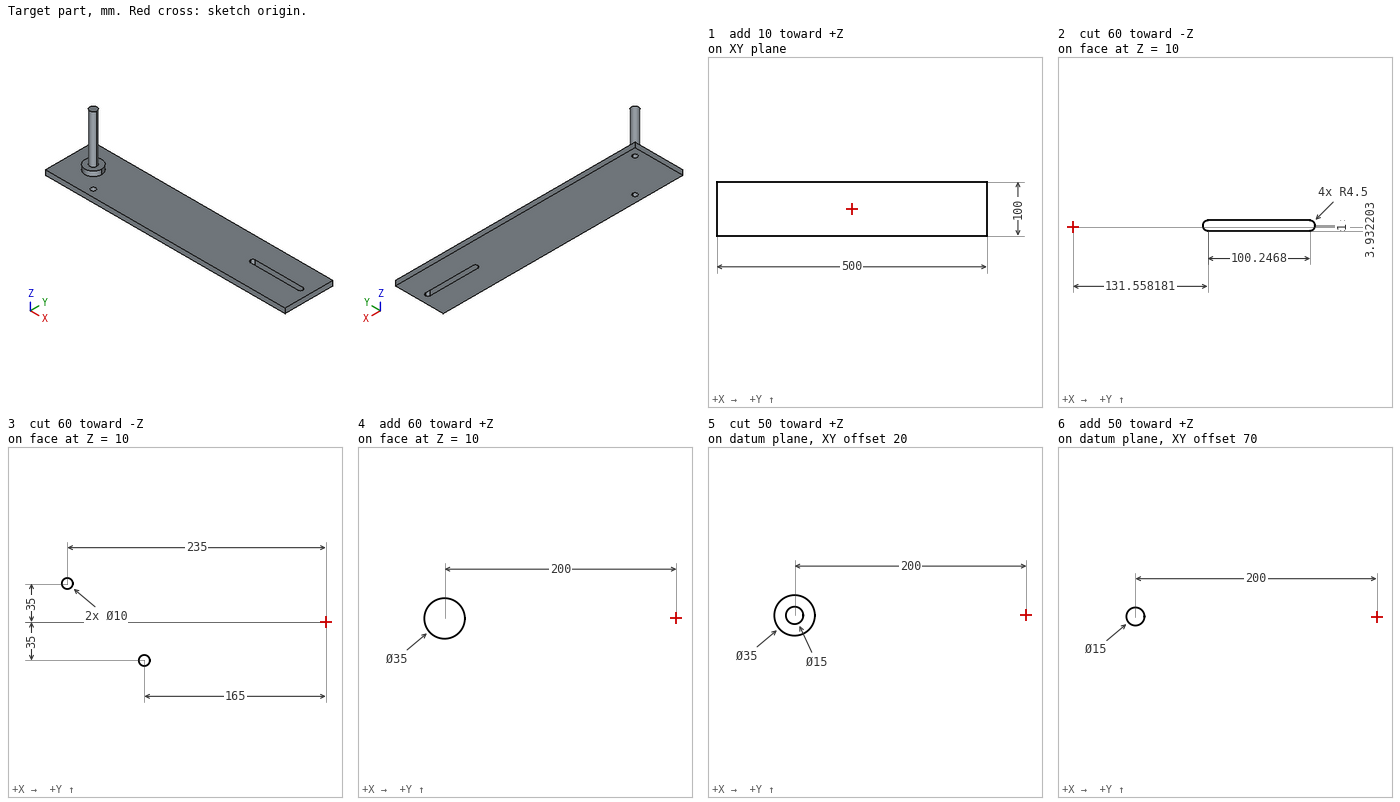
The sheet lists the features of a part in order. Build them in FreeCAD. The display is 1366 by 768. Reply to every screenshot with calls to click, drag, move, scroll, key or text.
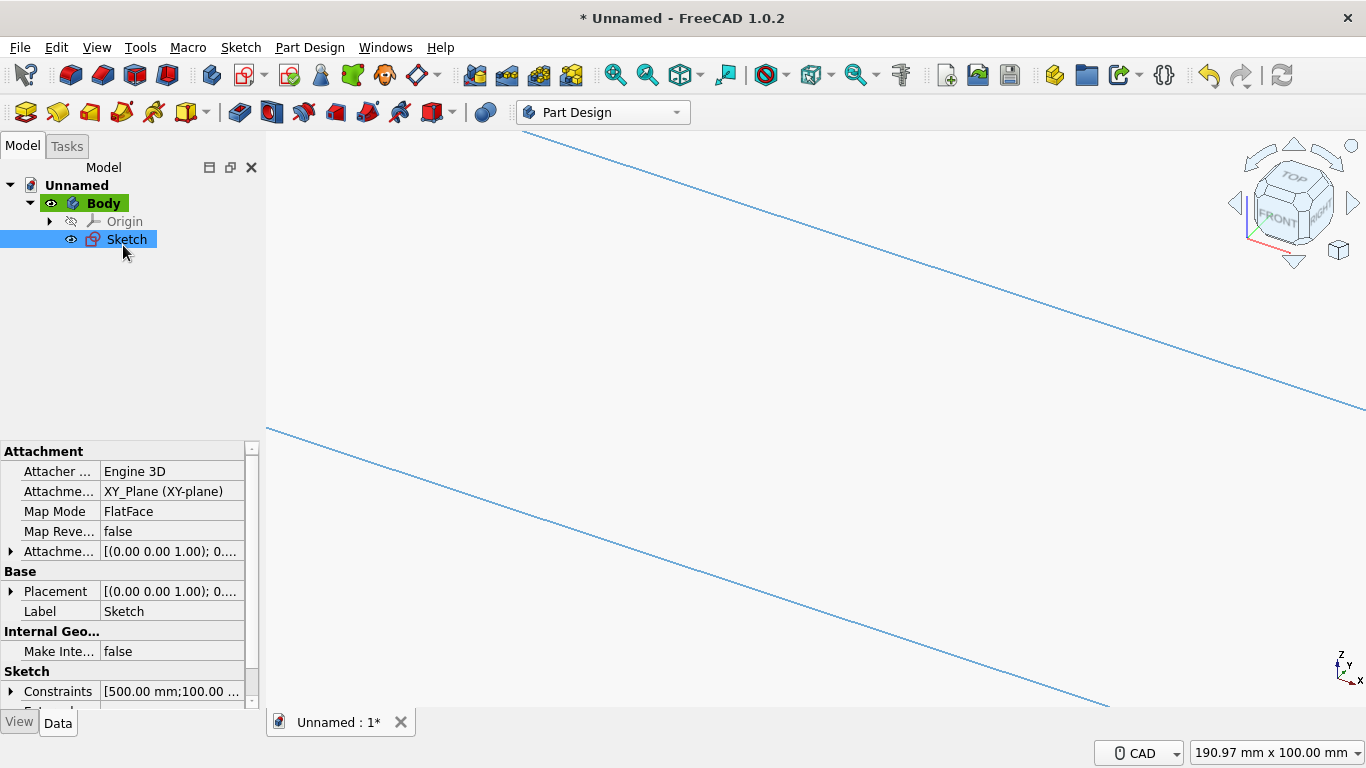
click(26, 112)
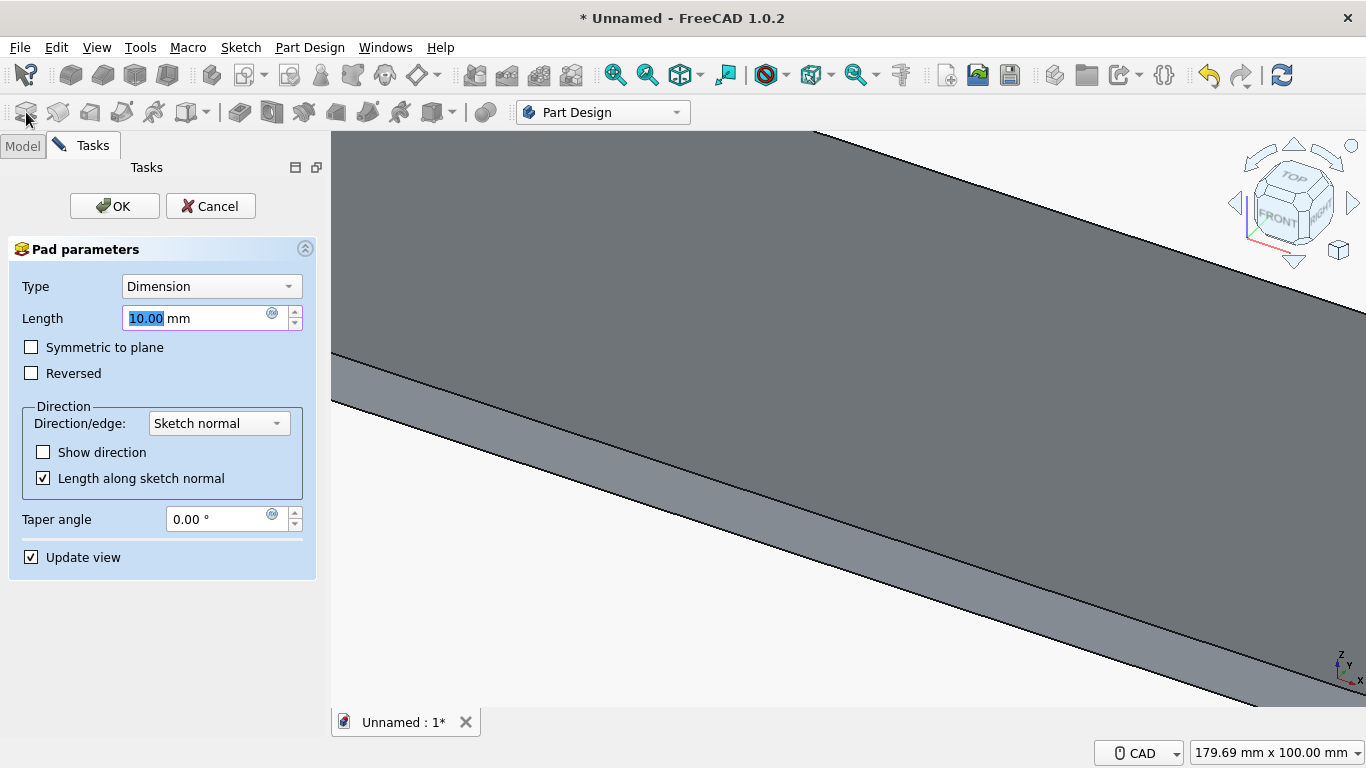
text(10)
key(Tab)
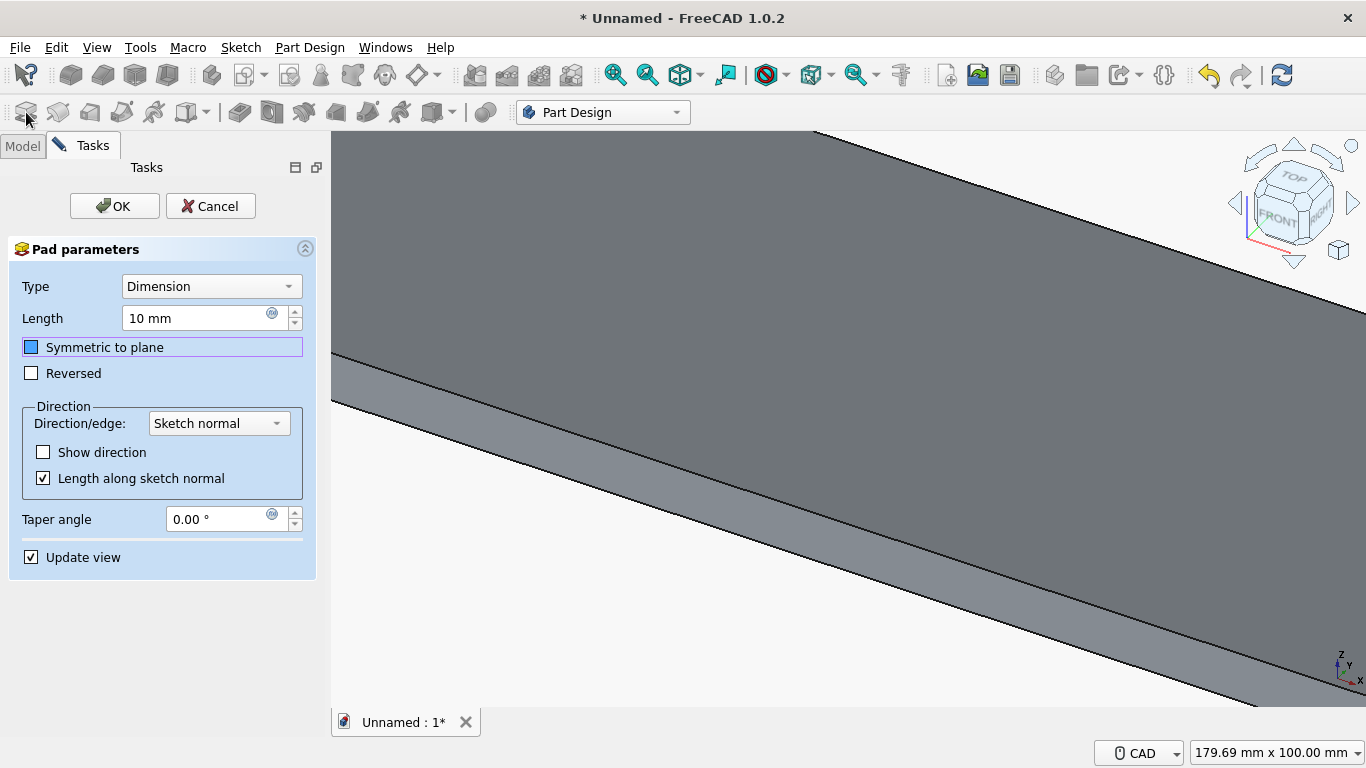
click(115, 206)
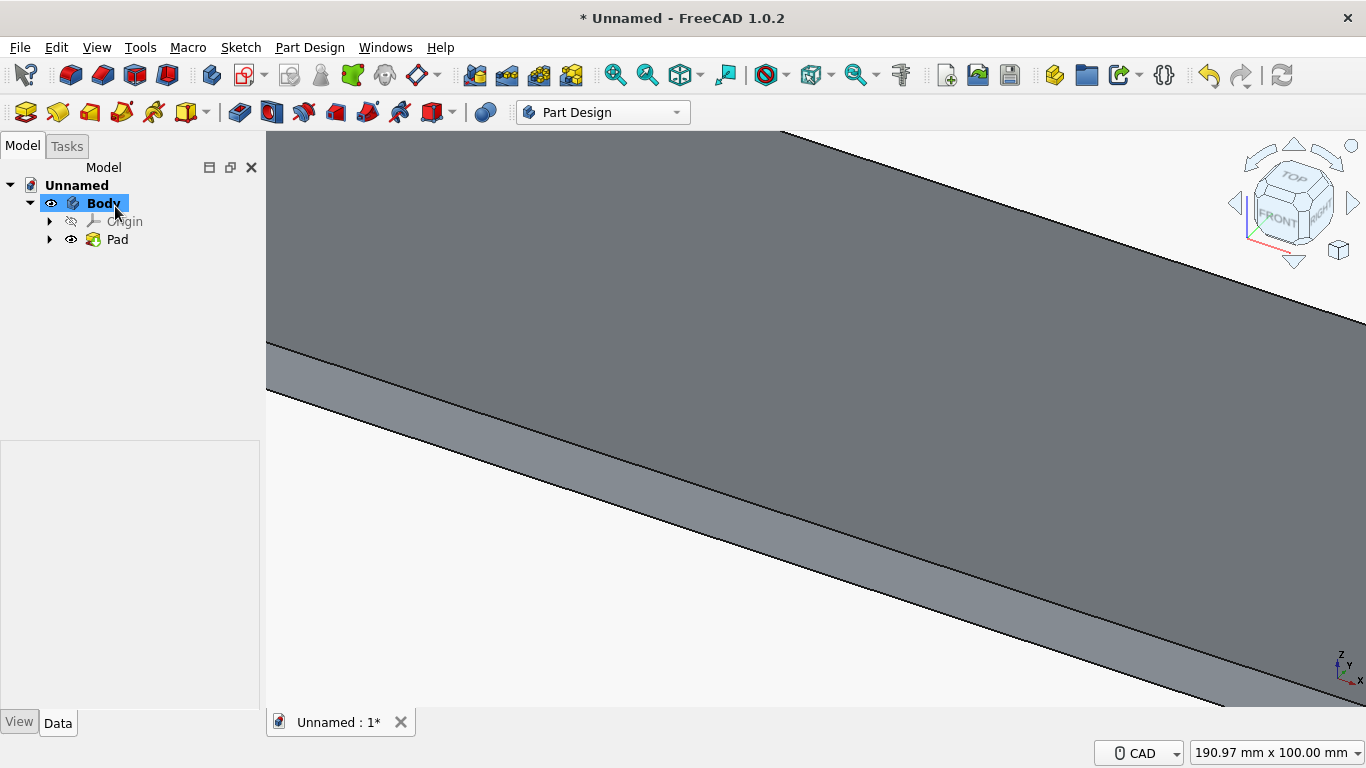
key(v)
key(f)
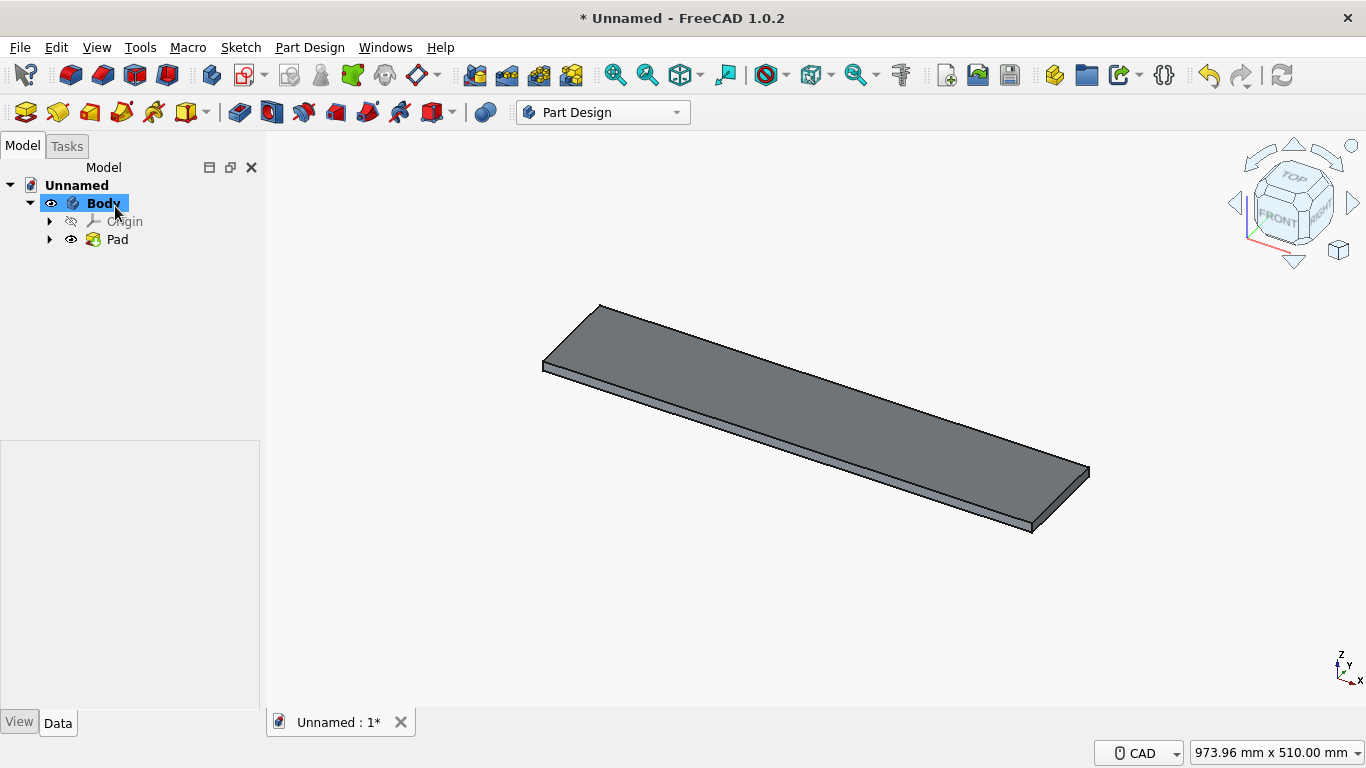
click(956, 460)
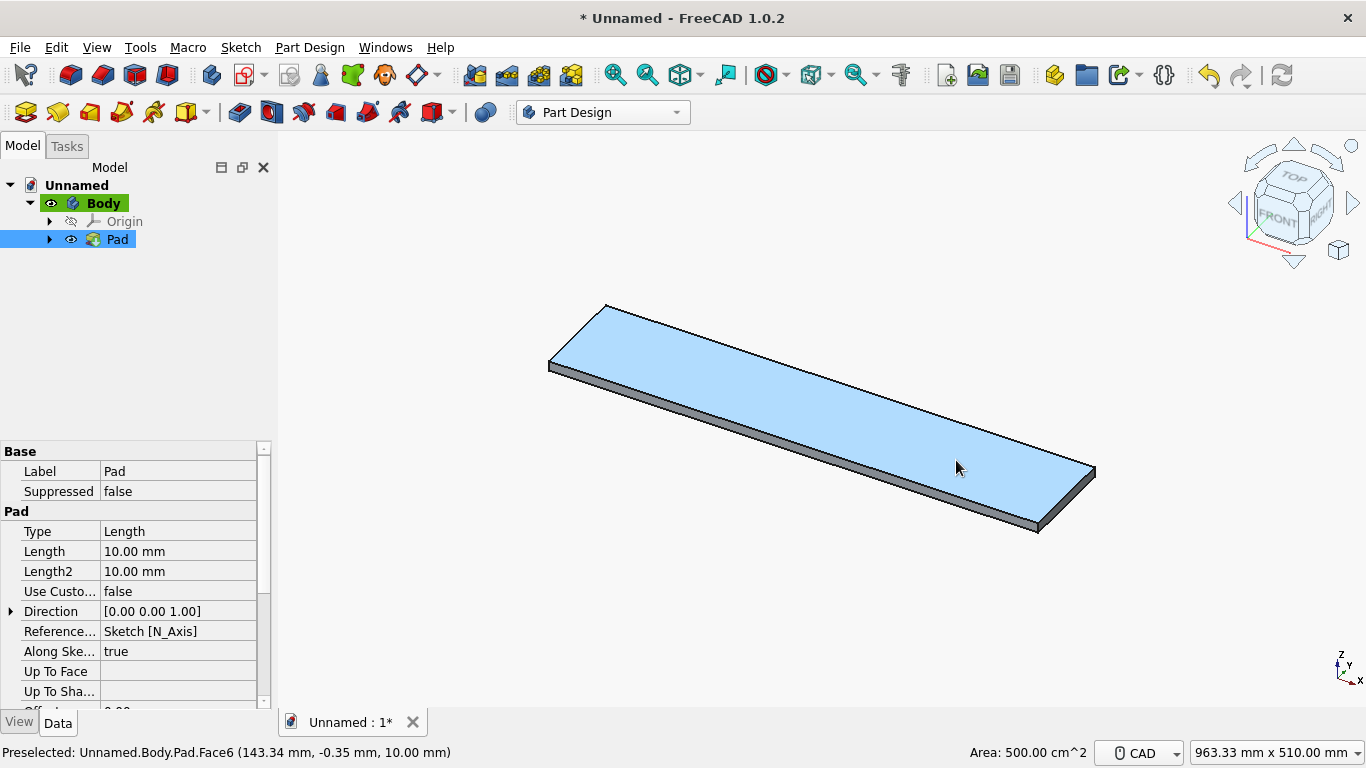
click(244, 76)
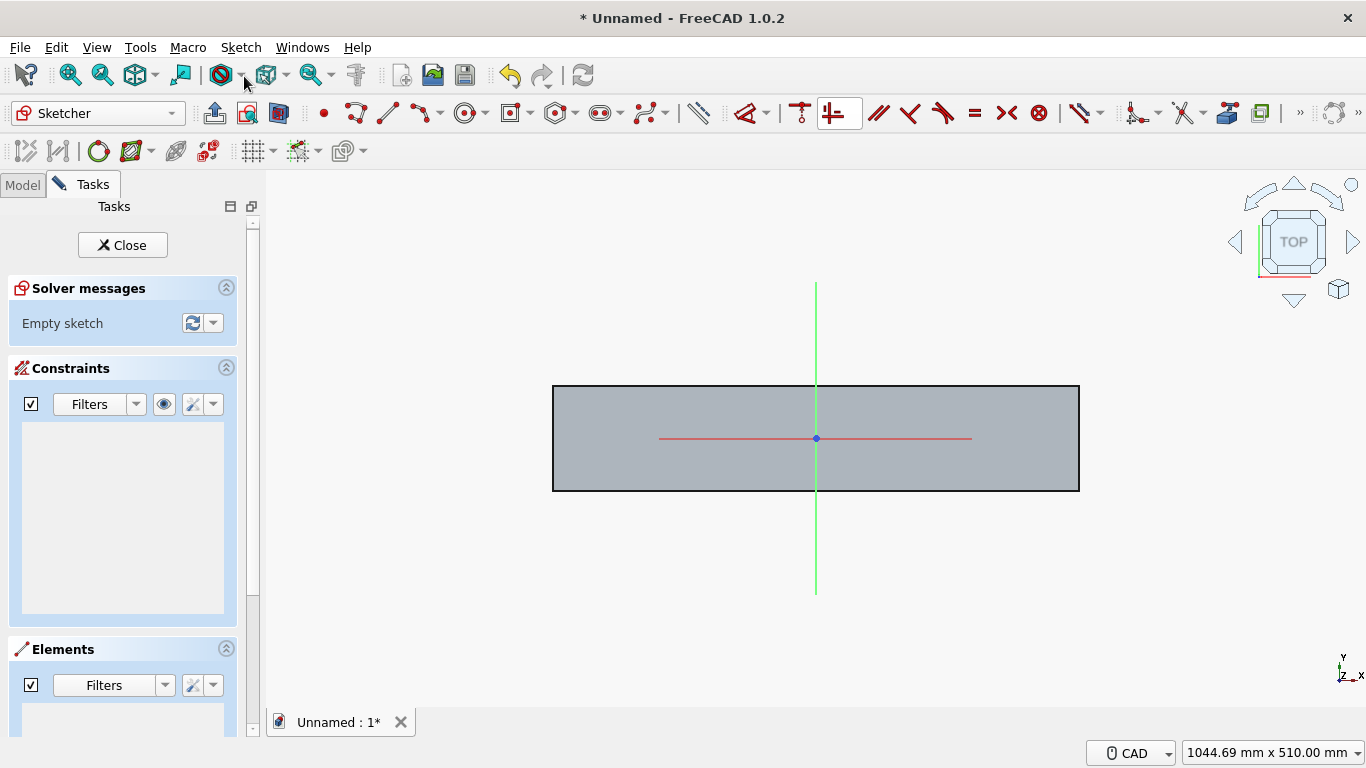
scroll(1053, 437, up, 5)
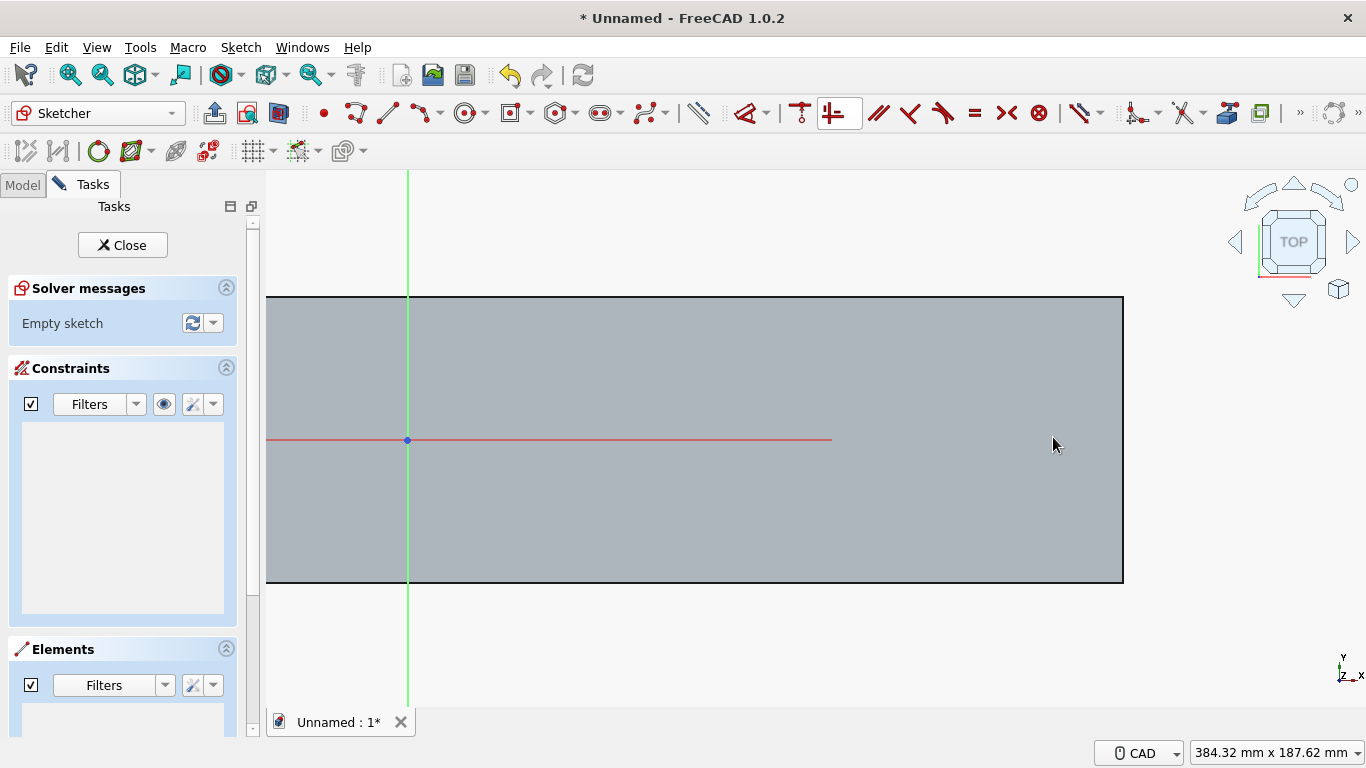
click(388, 114)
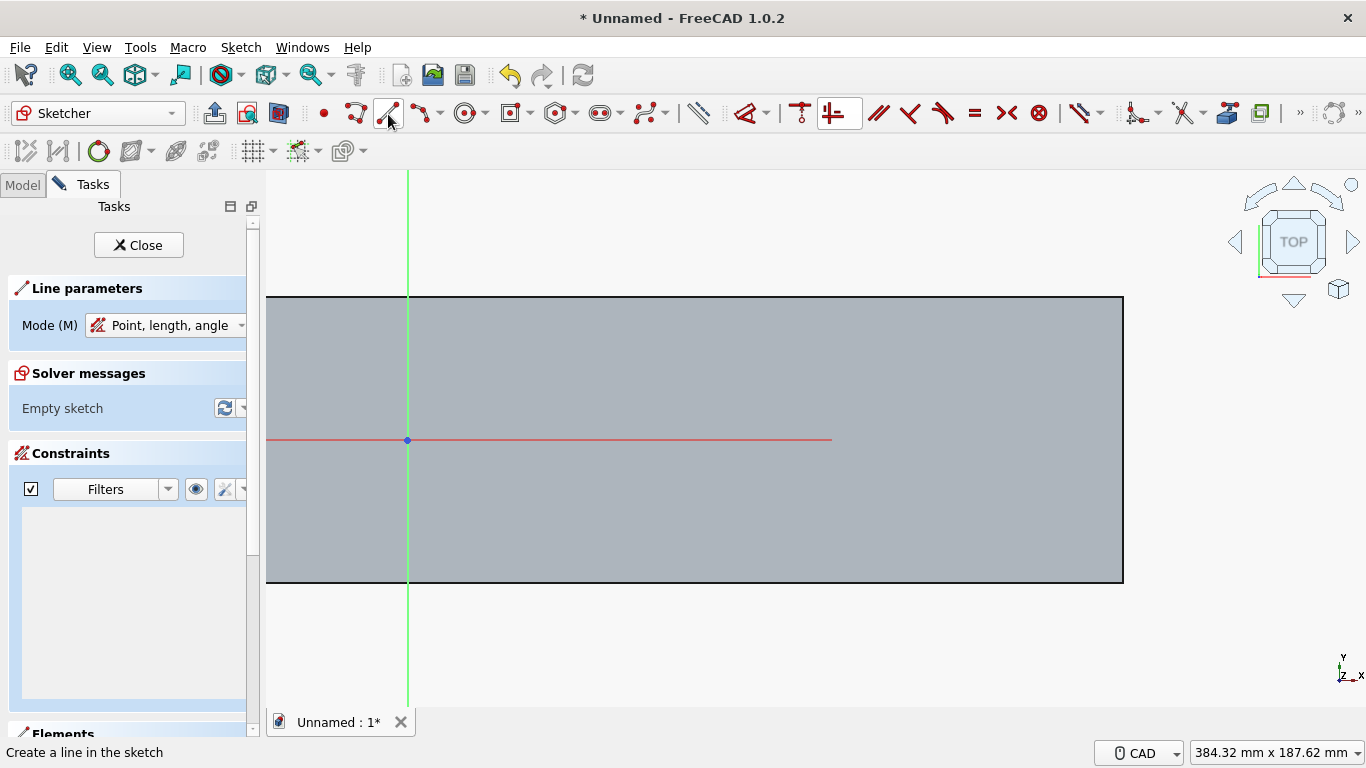
scroll(784, 451, up, 2)